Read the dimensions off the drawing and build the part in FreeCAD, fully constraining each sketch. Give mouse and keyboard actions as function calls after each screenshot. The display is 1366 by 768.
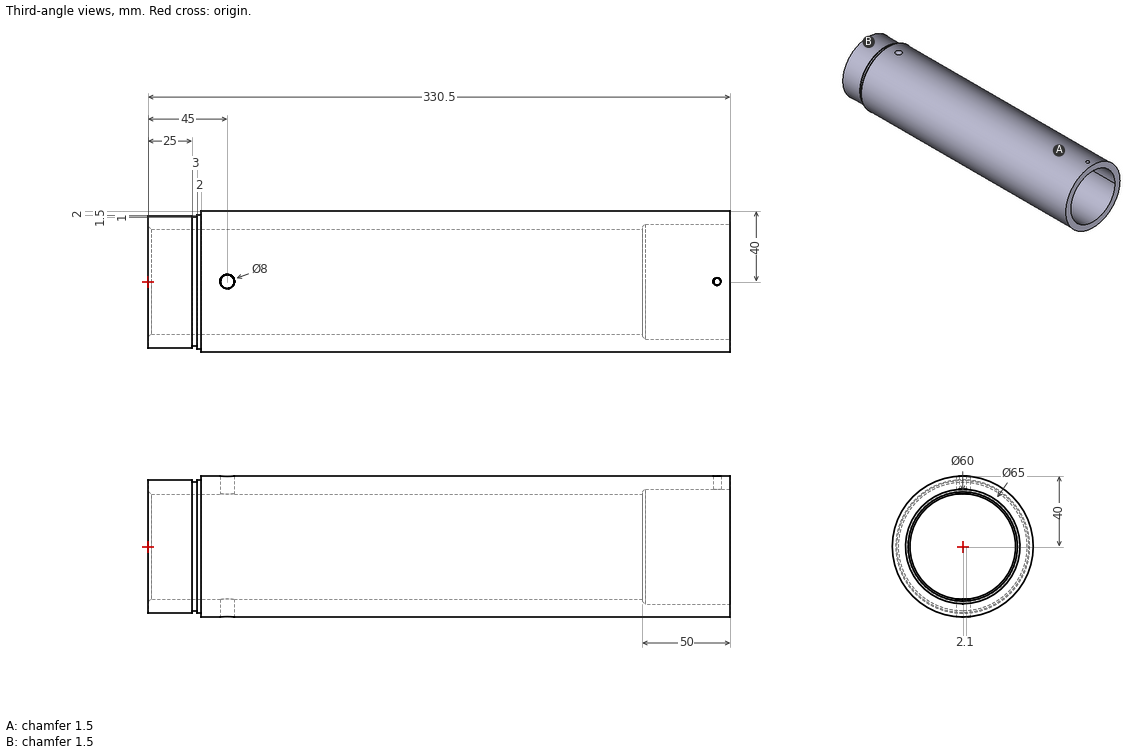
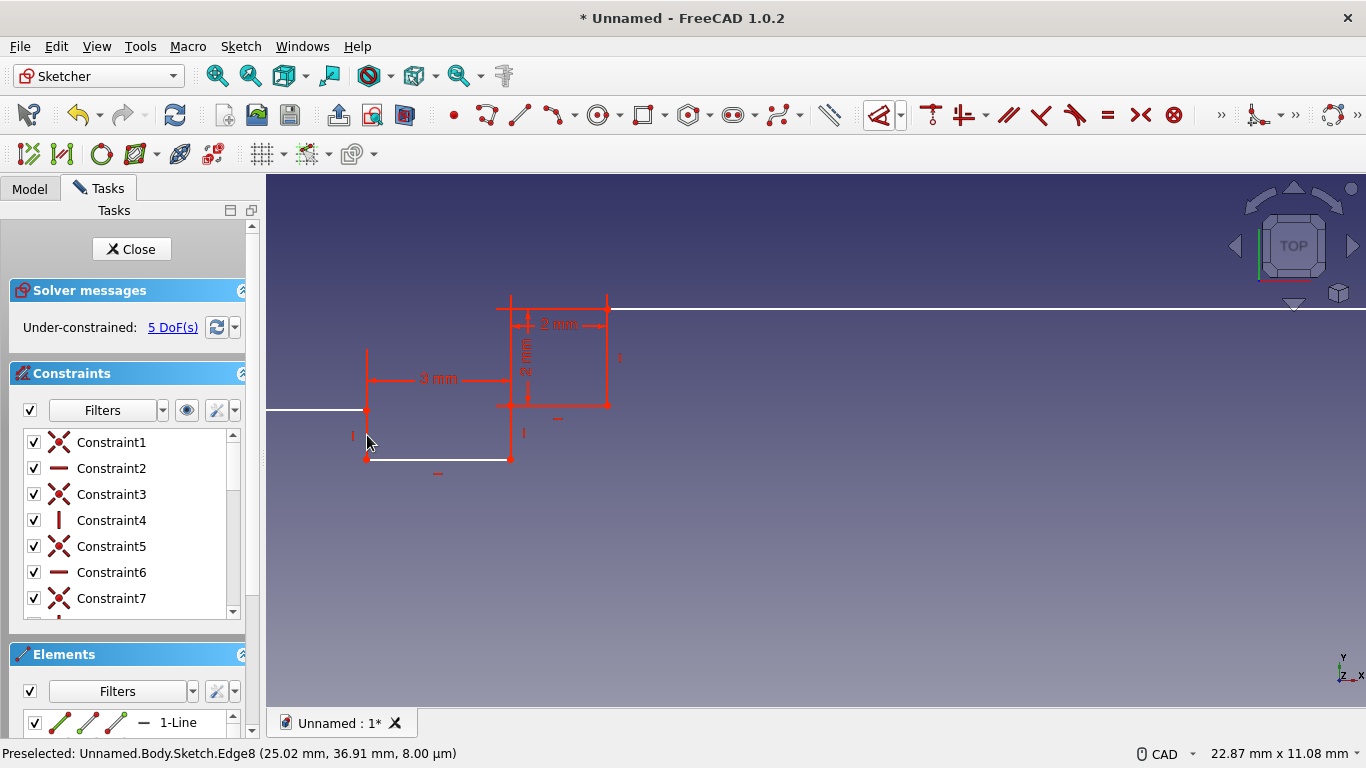
click(900, 116)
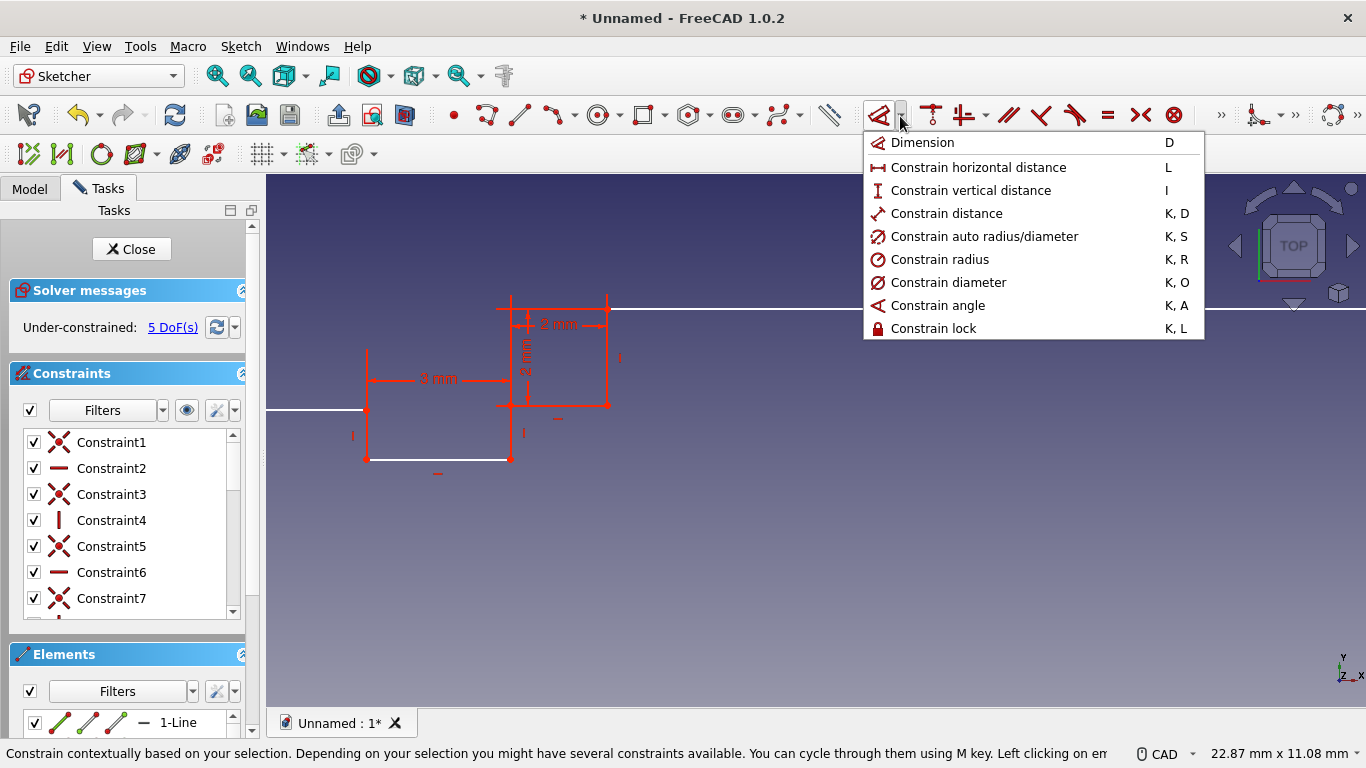
click(1034, 190)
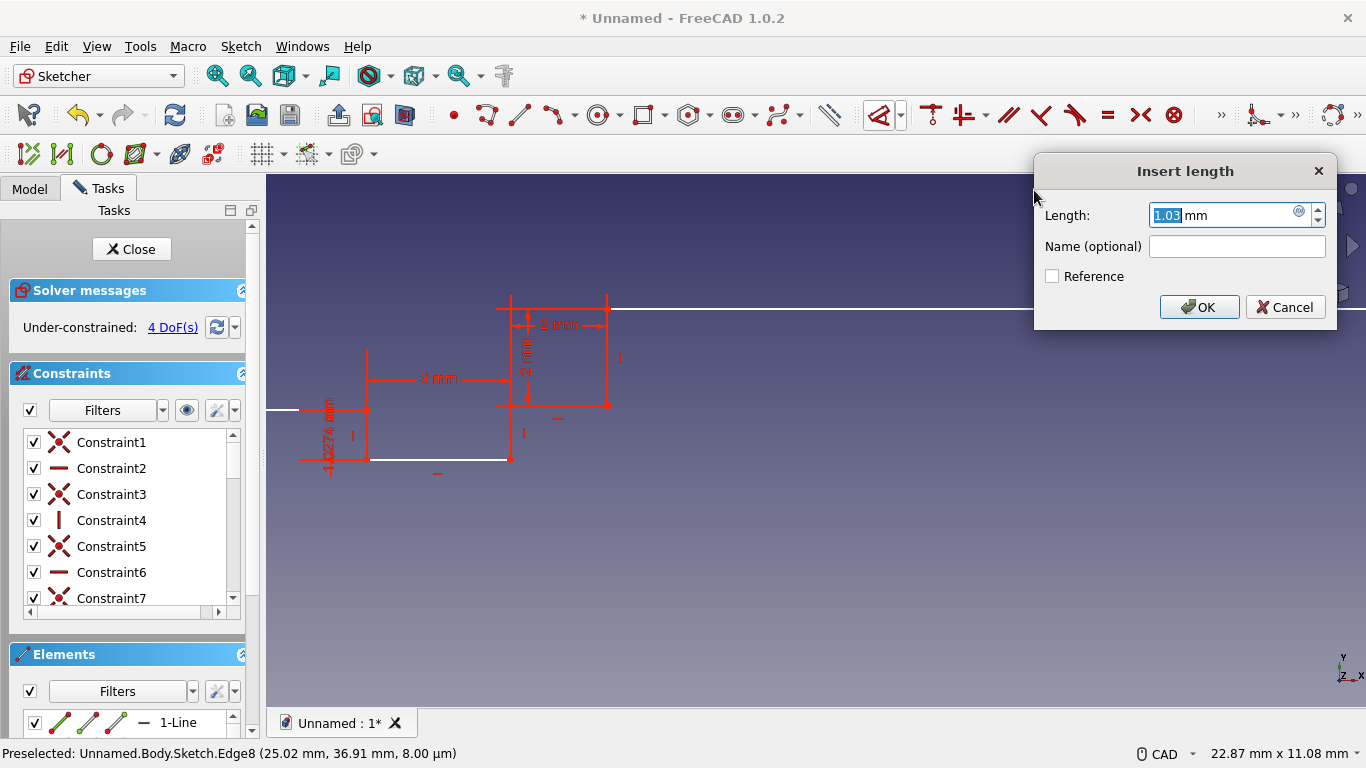
text(1)
key(Return)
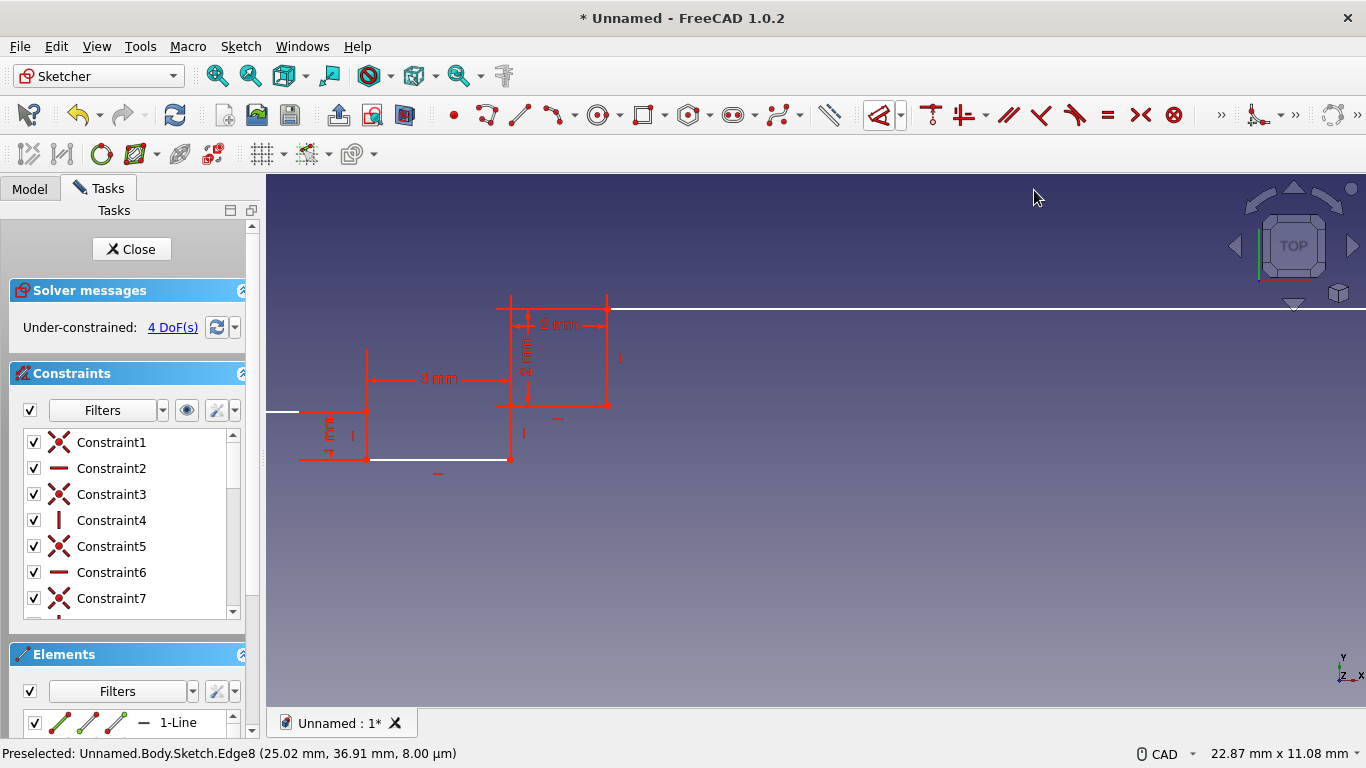
scroll(414, 398, down, 15)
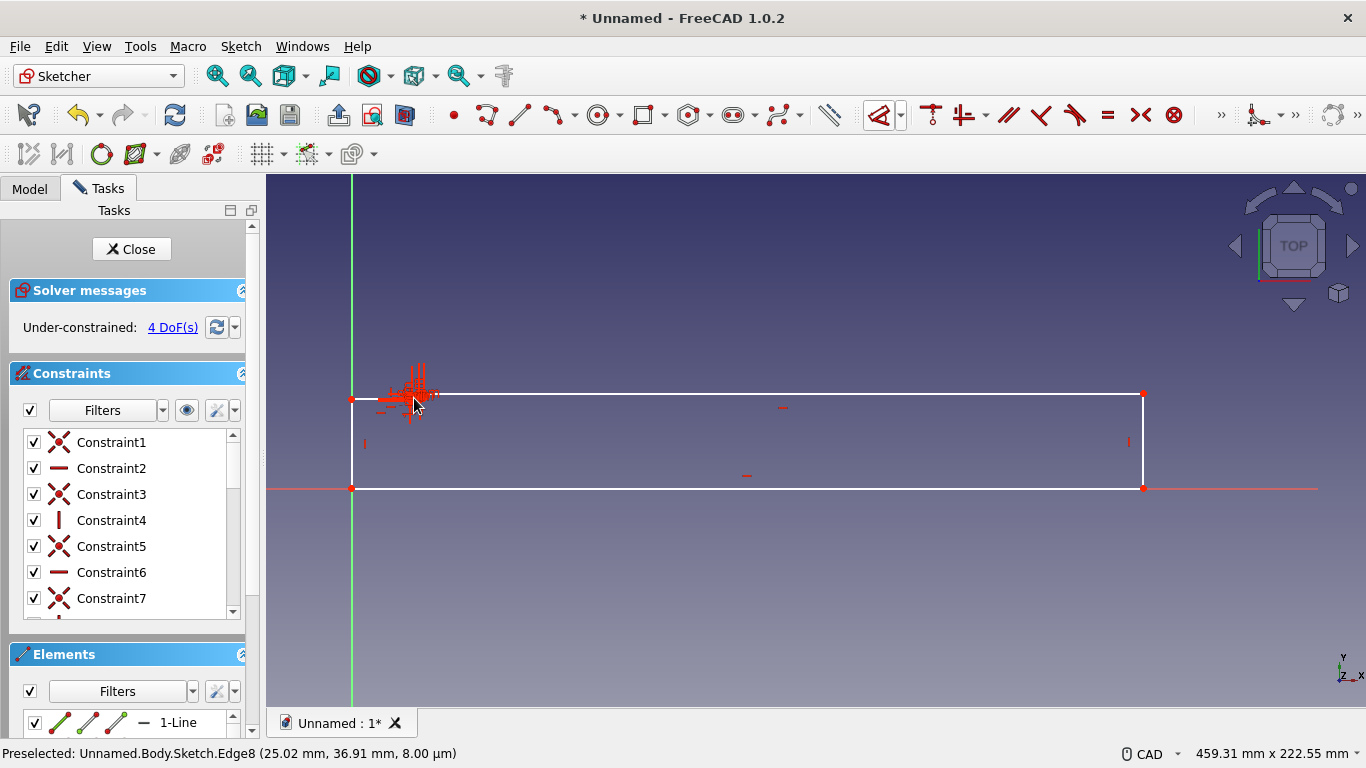
click(1143, 460)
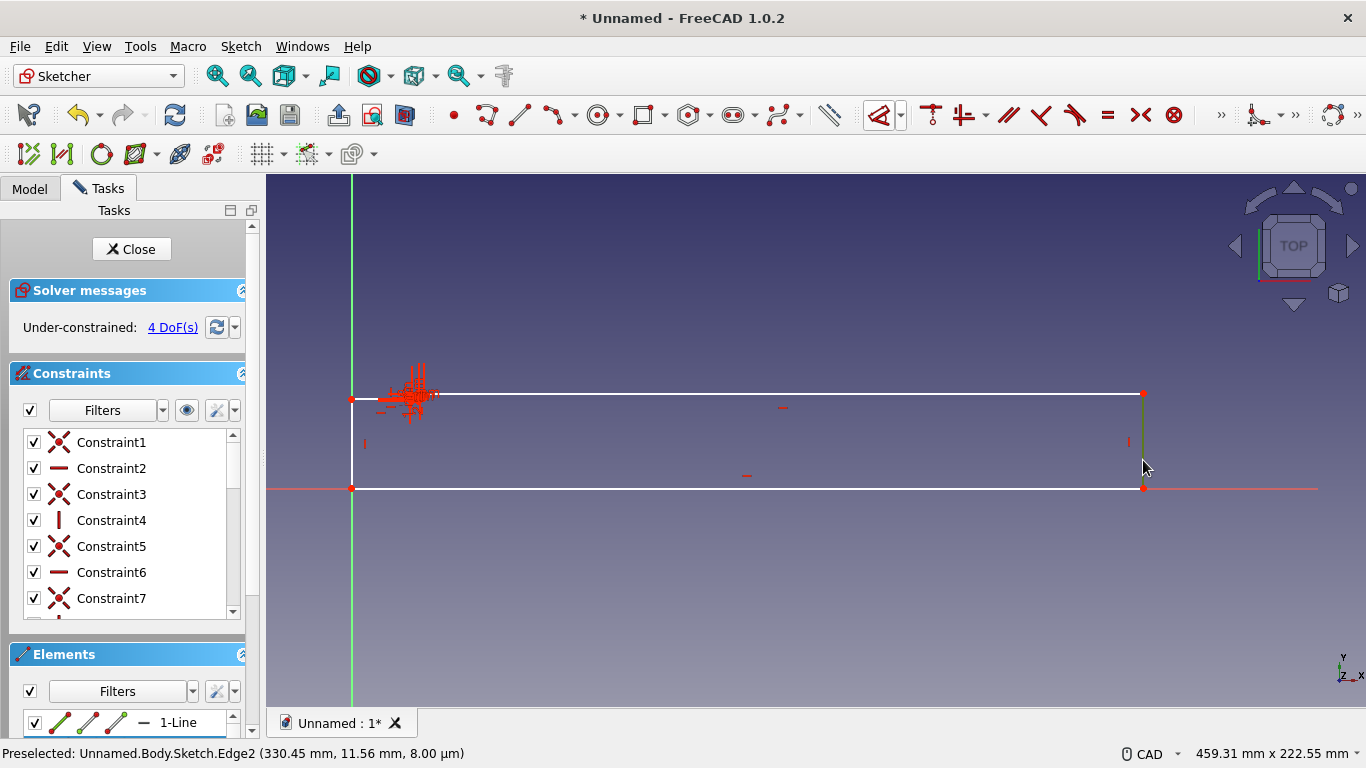
click(900, 116)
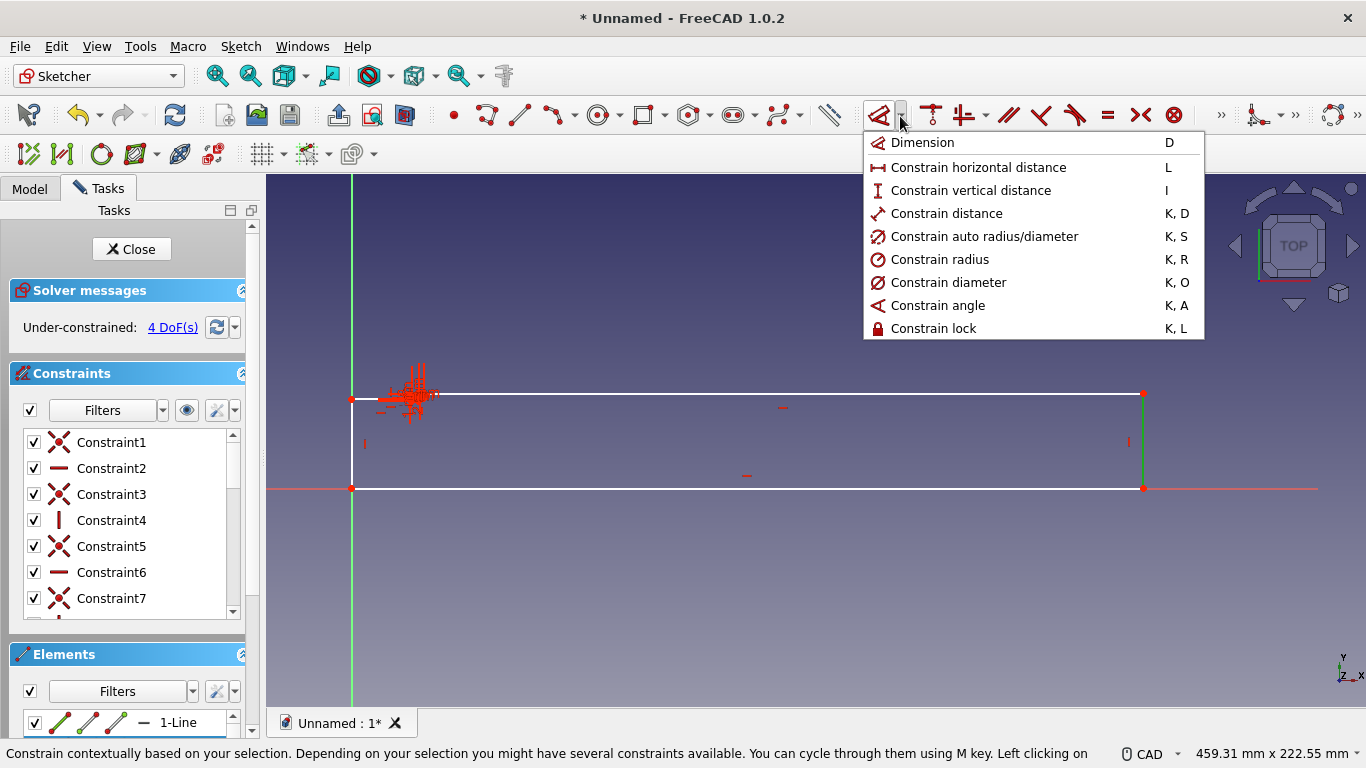
click(1034, 190)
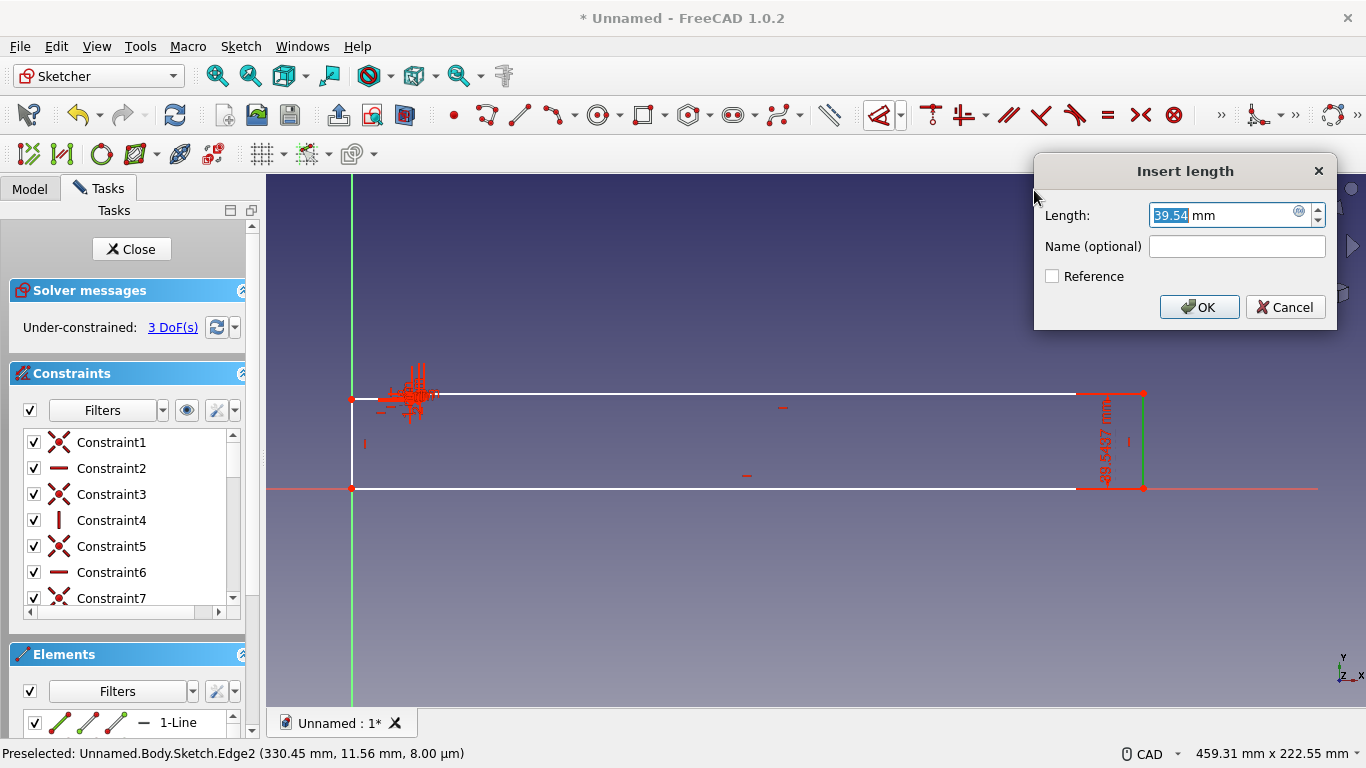
text(40)
key(Return)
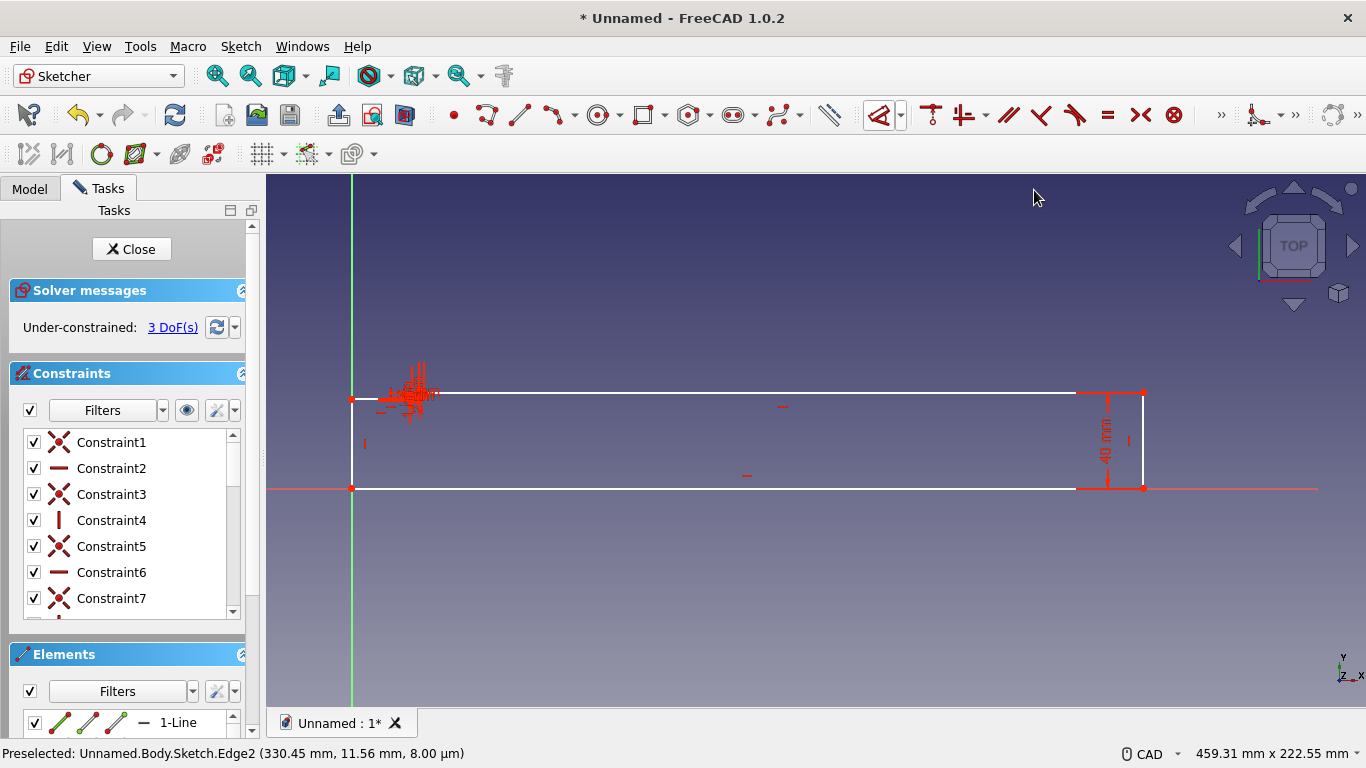
click(370, 399)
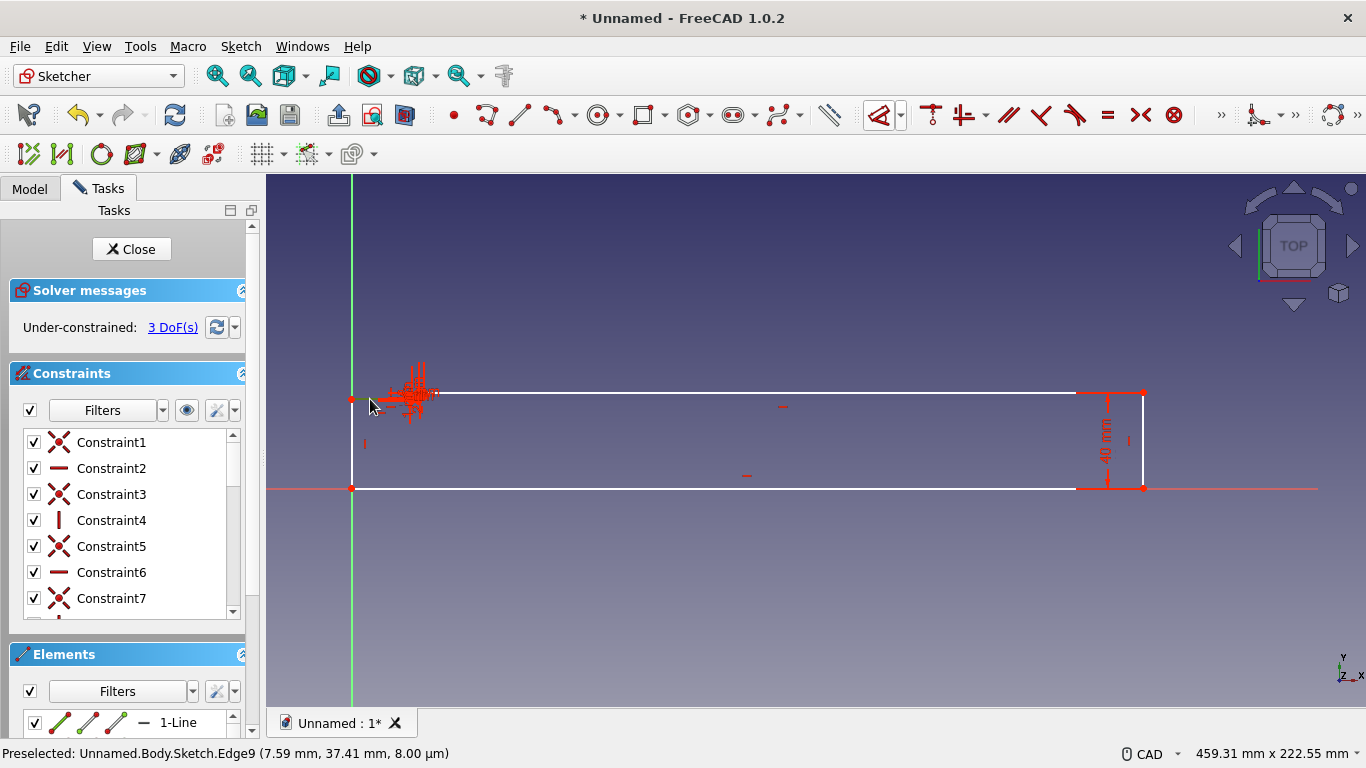
key(l)